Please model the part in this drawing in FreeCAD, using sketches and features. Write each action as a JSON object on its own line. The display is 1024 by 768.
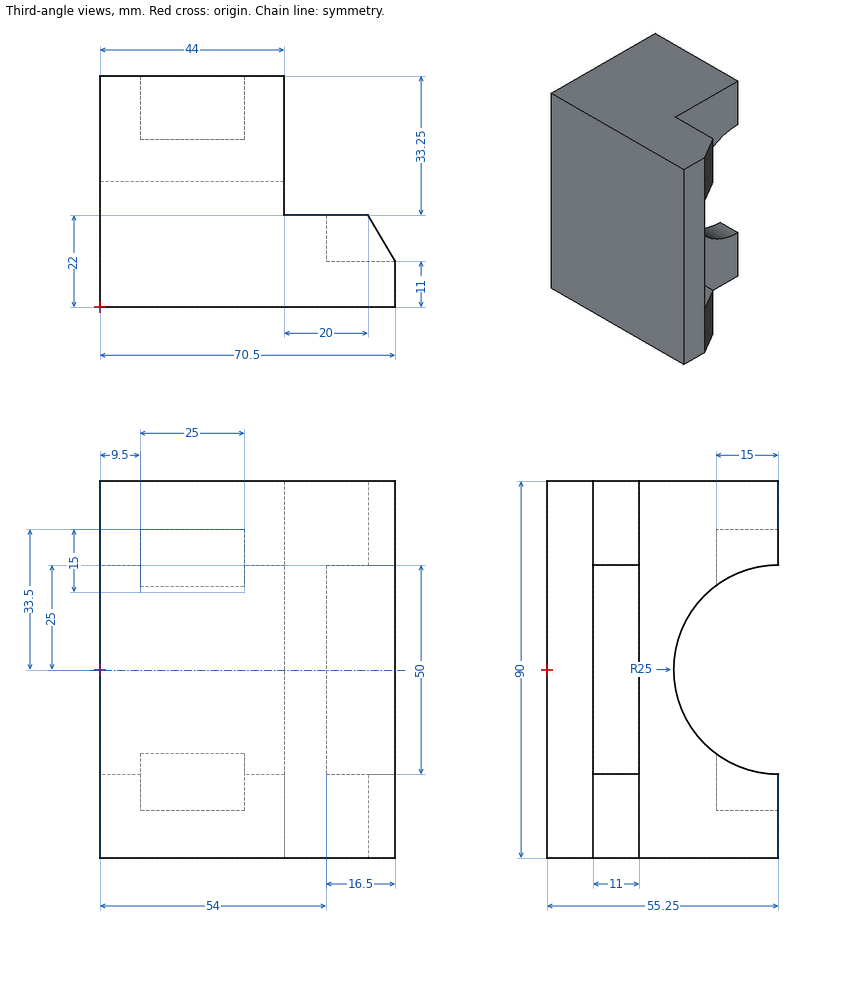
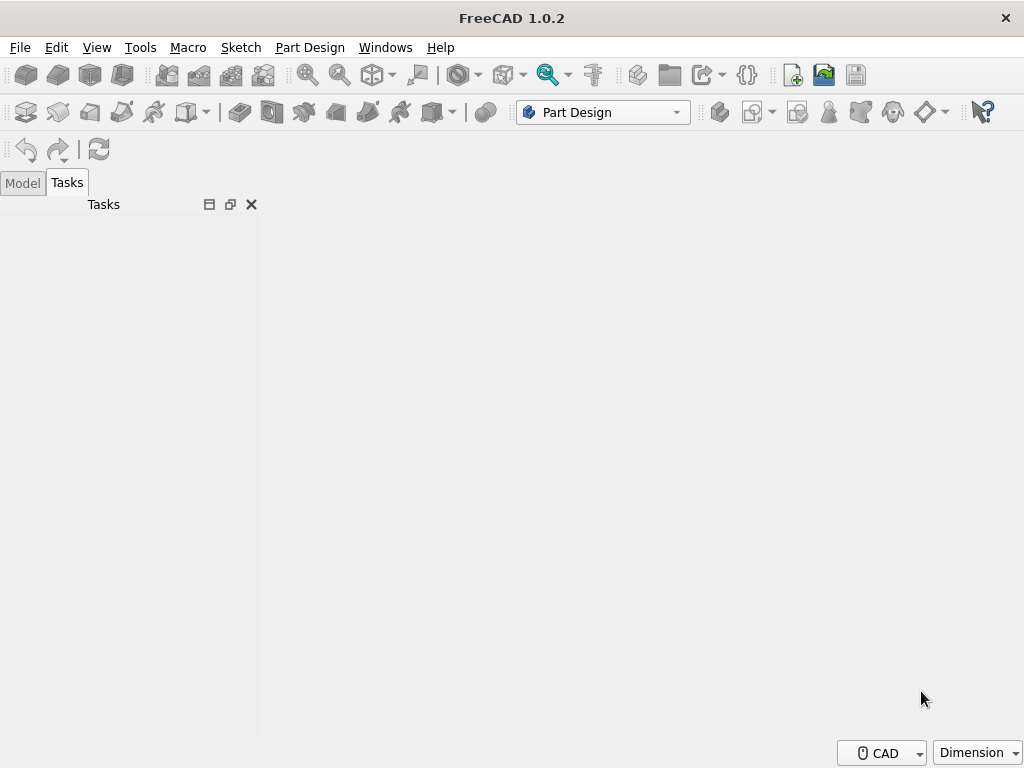
{"action": "left_click", "coordinate": [792, 76]}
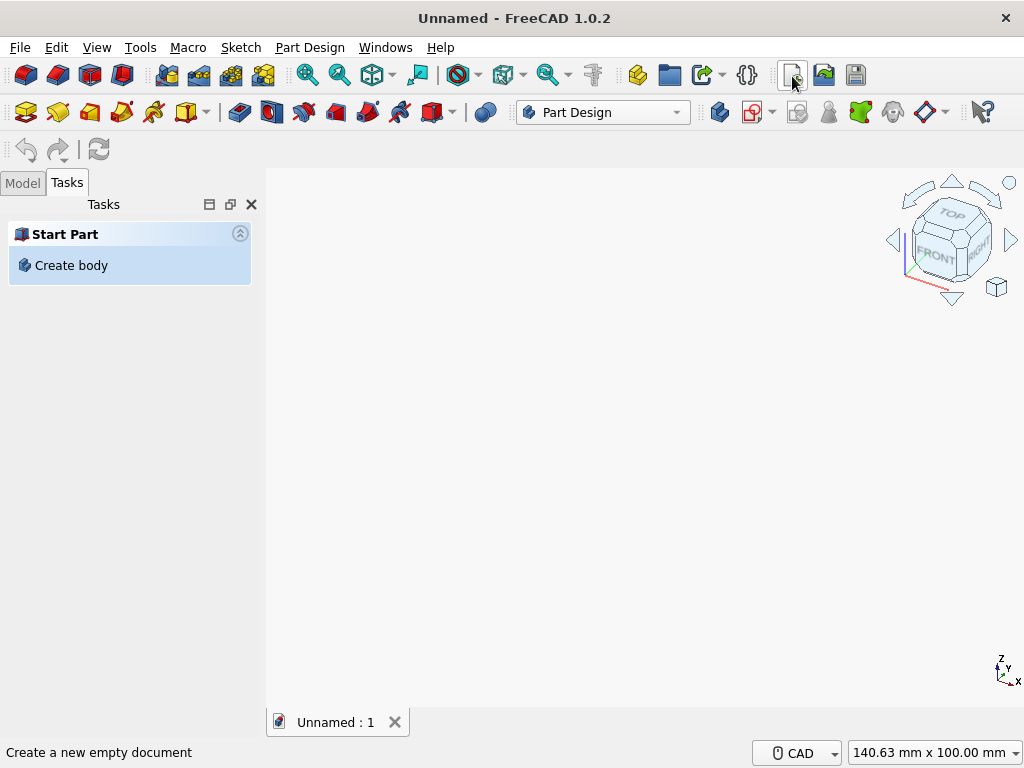
{"action": "left_click", "coordinate": [752, 112]}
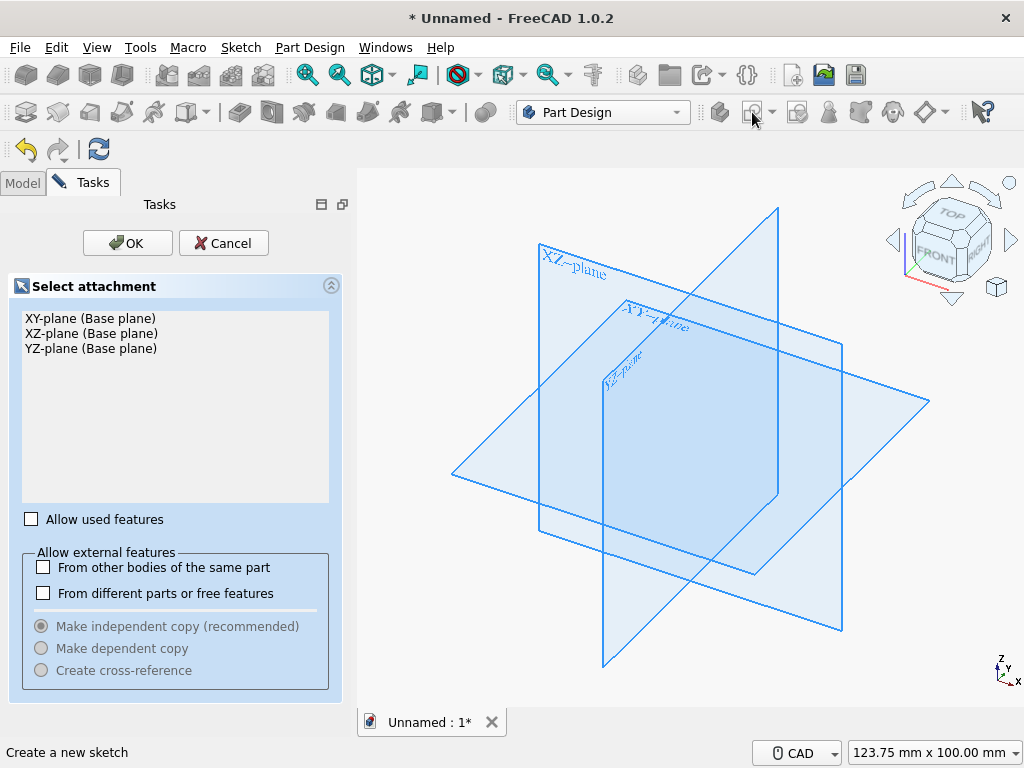
{"action": "left_click", "coordinate": [82, 318]}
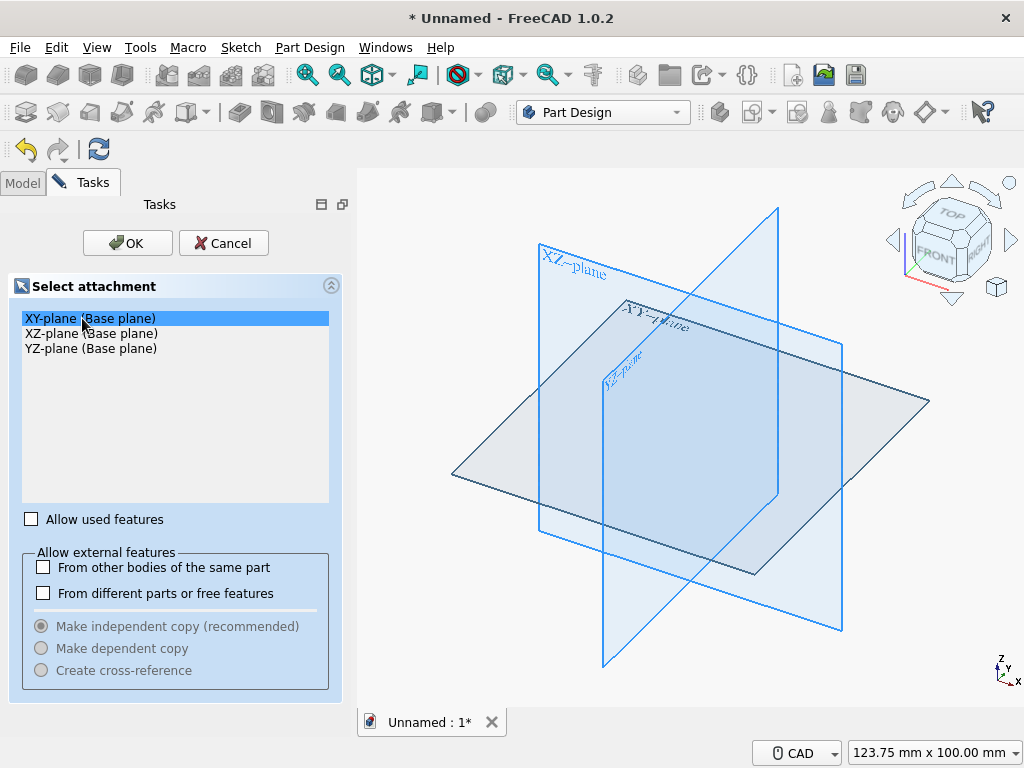
{"action": "left_click", "coordinate": [128, 243]}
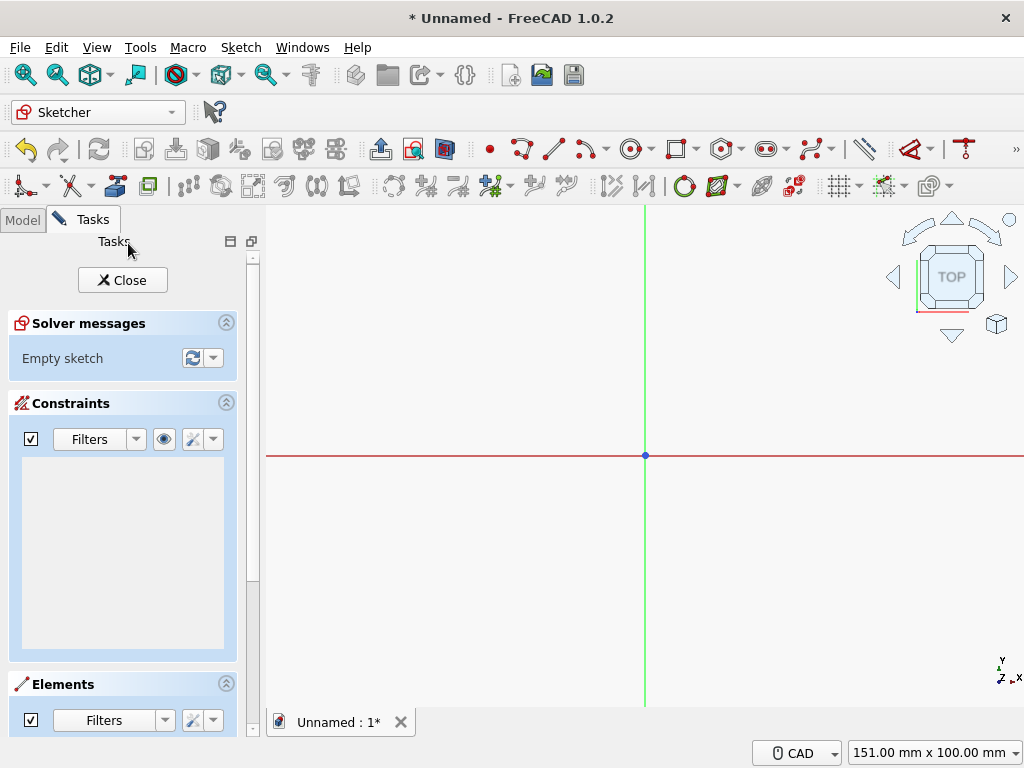
{"action": "scroll", "coordinate": [294, 679], "scroll_direction": "down", "scroll_amount": 2}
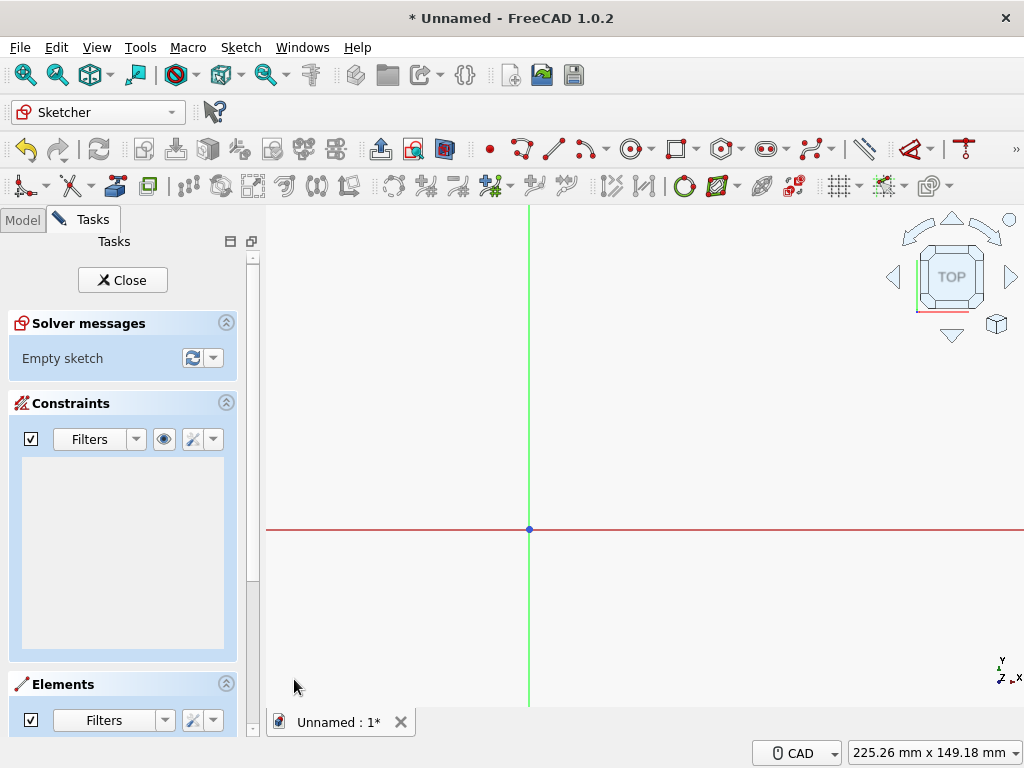
{"action": "scroll", "coordinate": [735, 414], "scroll_direction": "up", "scroll_amount": 3}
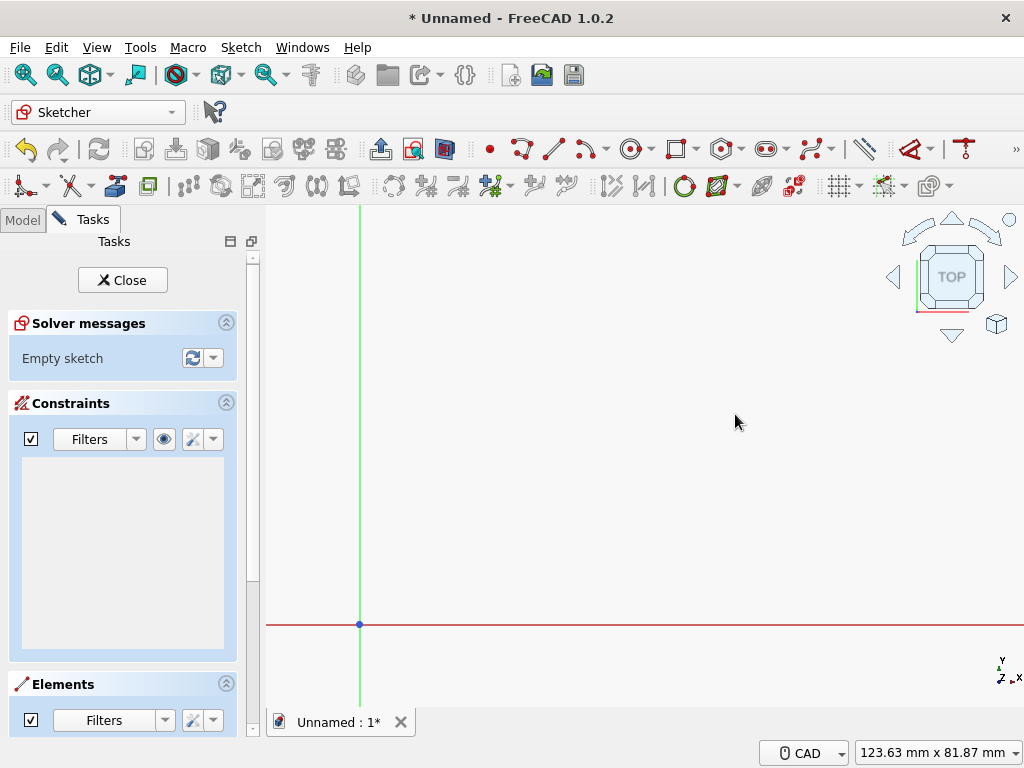
{"action": "key", "text": "g m"}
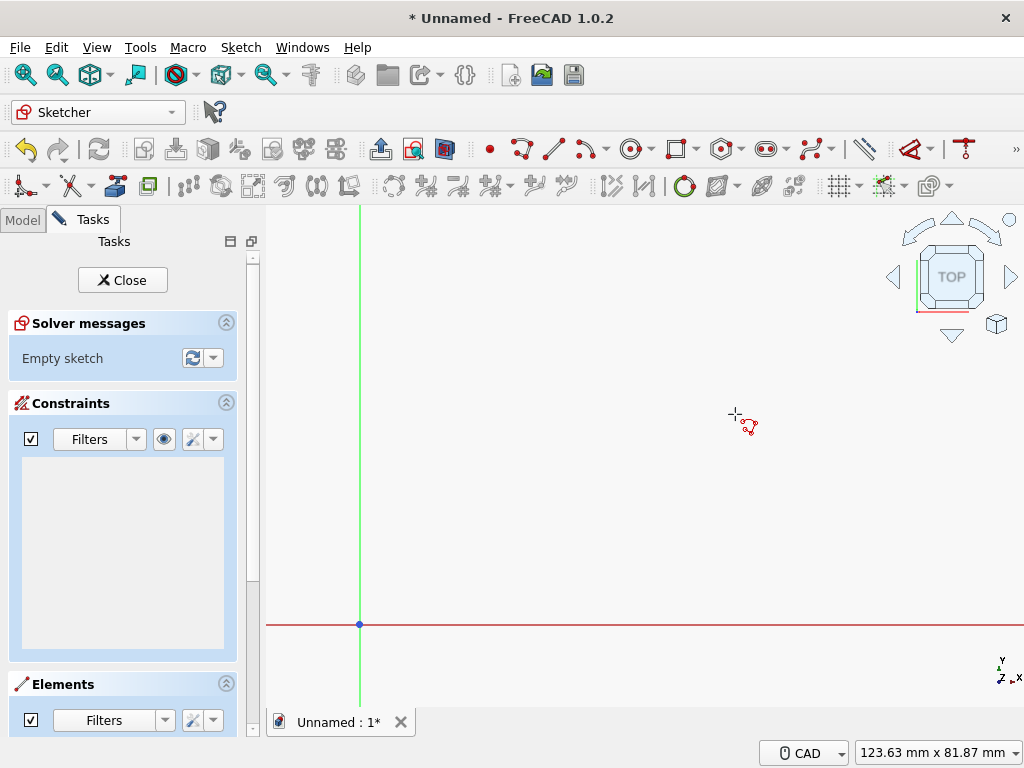
{"action": "left_click", "coordinate": [360, 625]}
{"action": "left_click", "coordinate": [792, 616]}
{"action": "left_click", "coordinate": [792, 557]}
{"action": "left_click", "coordinate": [752, 490]}
{"action": "left_click", "coordinate": [629, 490]}
{"action": "left_click", "coordinate": [629, 286]}
{"action": "left_click", "coordinate": [369, 286]}
{"action": "left_click", "coordinate": [360, 625]}
{"action": "key", "text": "Escape"}
{"action": "key", "text": "Escape"}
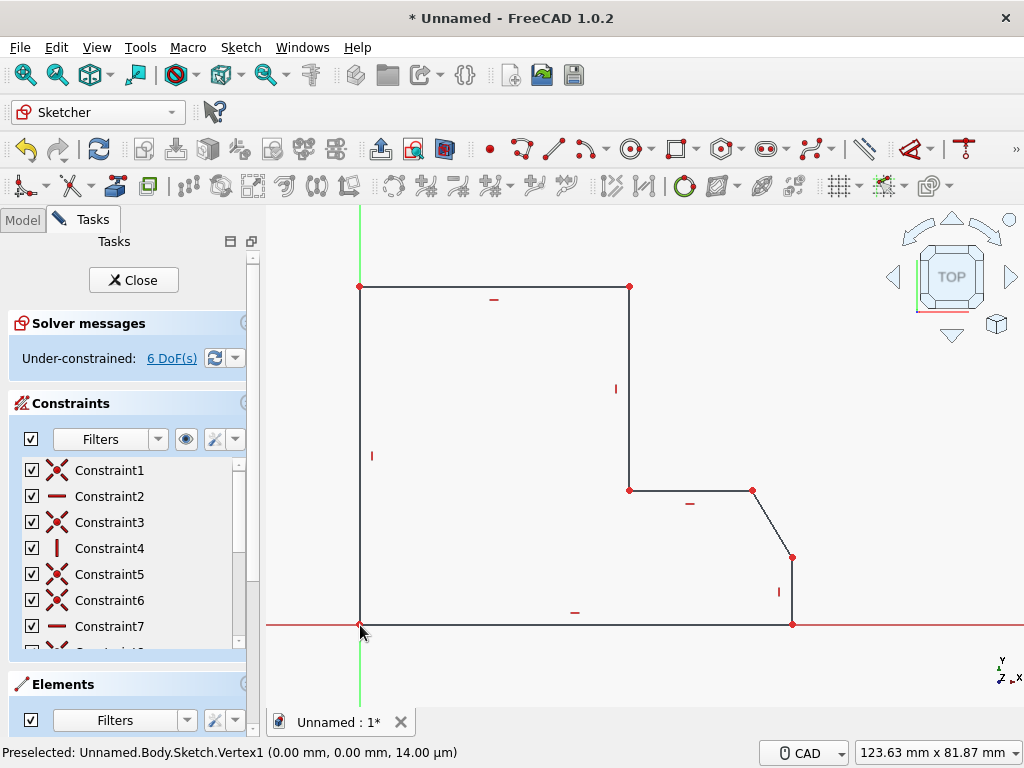
{"action": "left_click", "coordinate": [910, 150]}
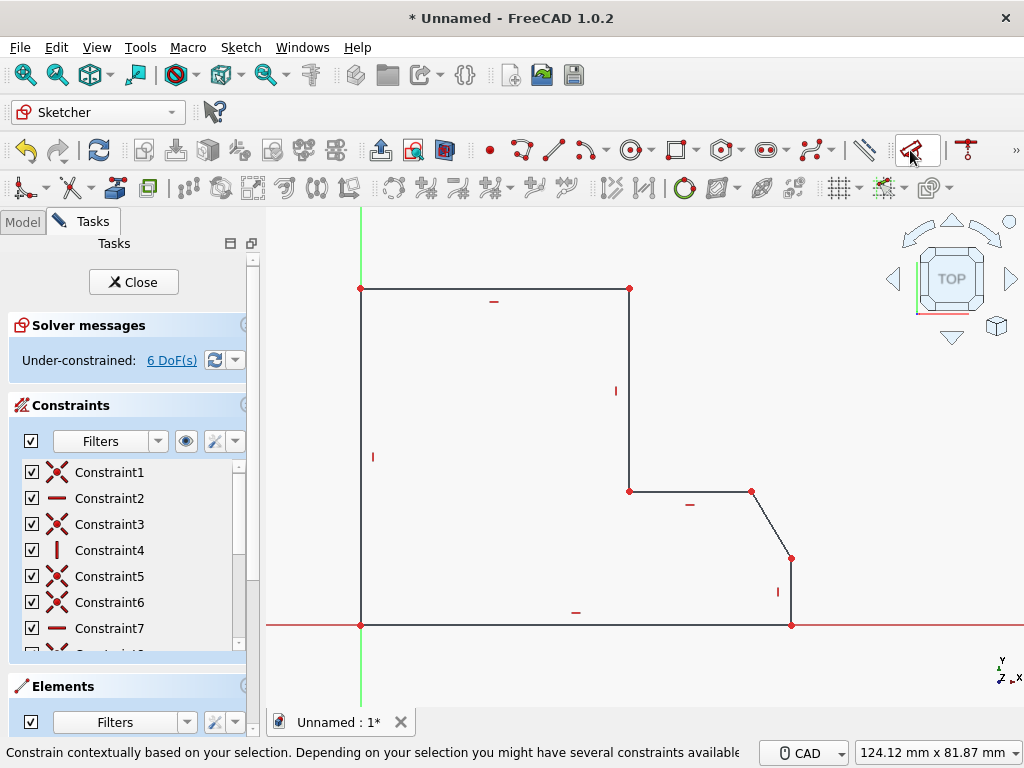
{"action": "left_click", "coordinate": [791, 605]}
{"action": "left_click", "coordinate": [825, 592]}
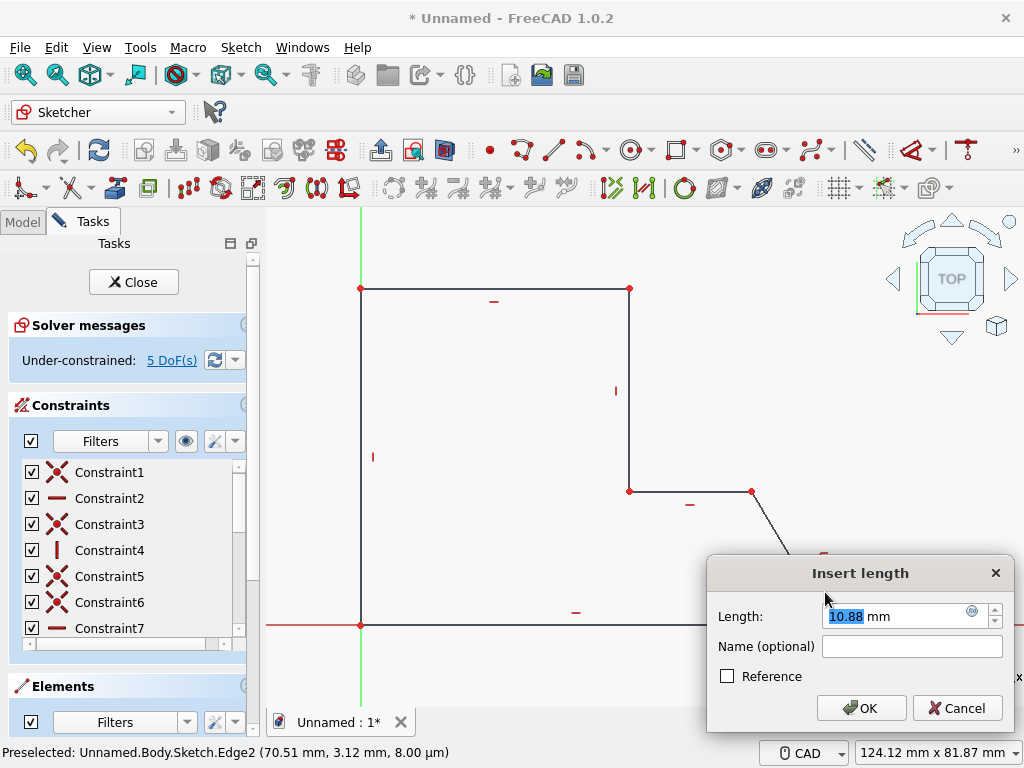
{"action": "type", "text": "11"}
{"action": "key", "text": "Return"}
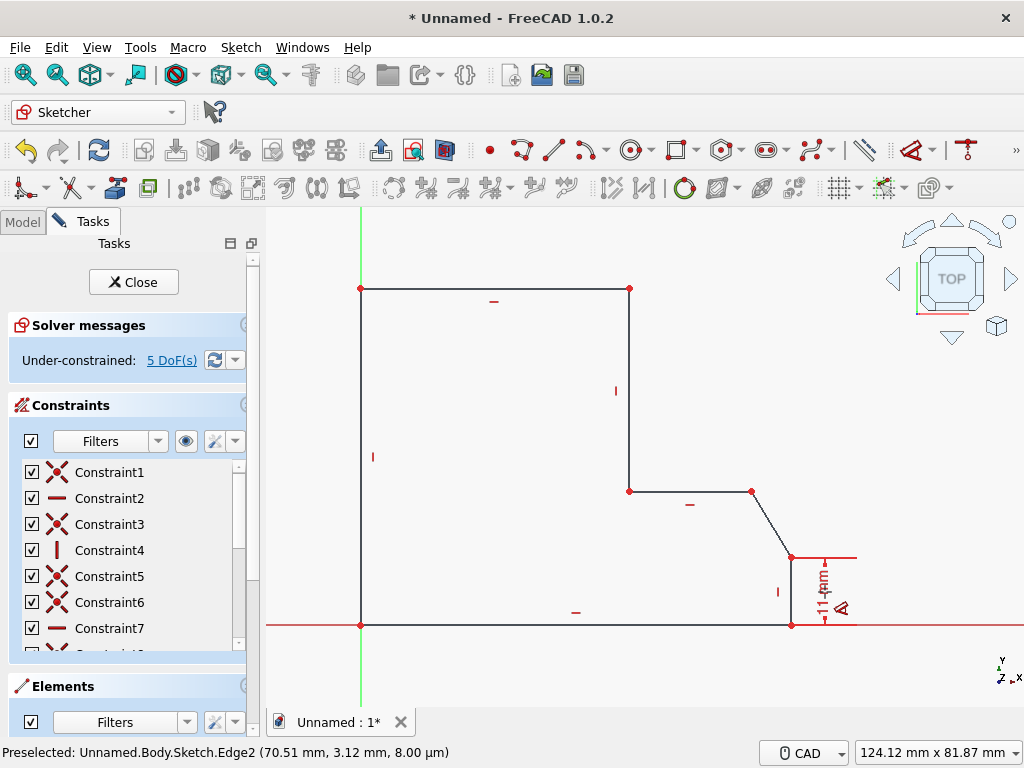
{"action": "left_click", "coordinate": [715, 492]}
{"action": "left_click", "coordinate": [690, 526]}